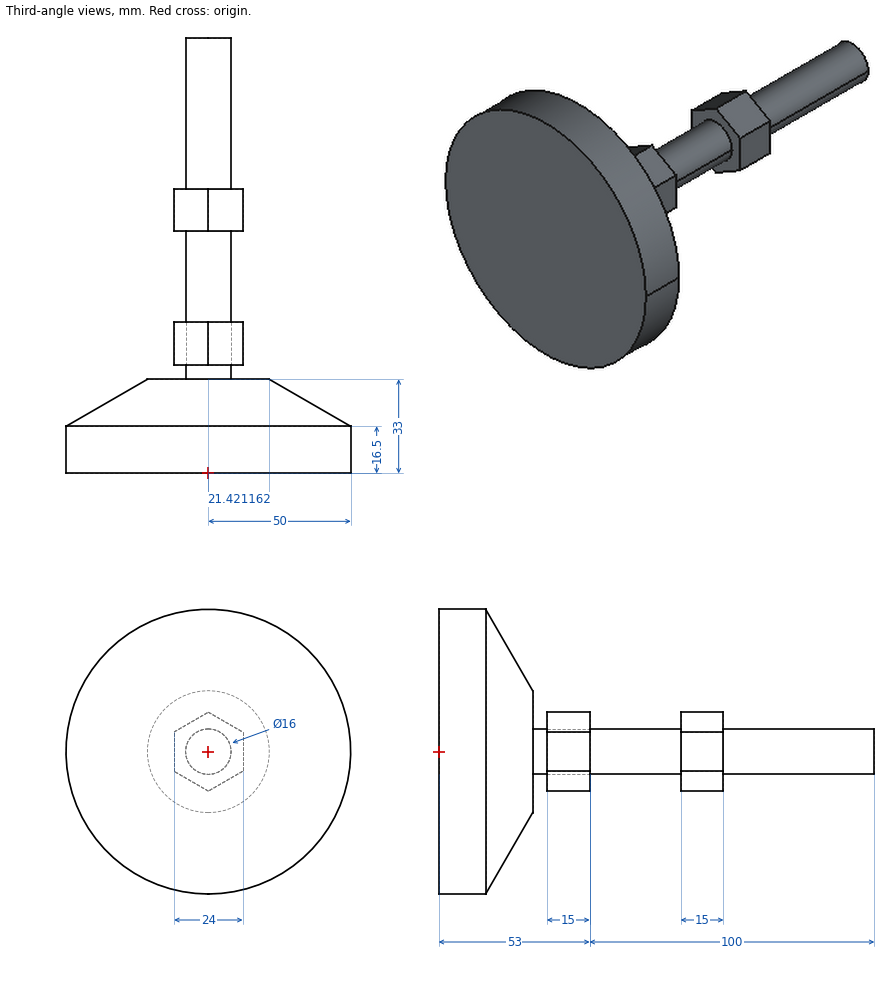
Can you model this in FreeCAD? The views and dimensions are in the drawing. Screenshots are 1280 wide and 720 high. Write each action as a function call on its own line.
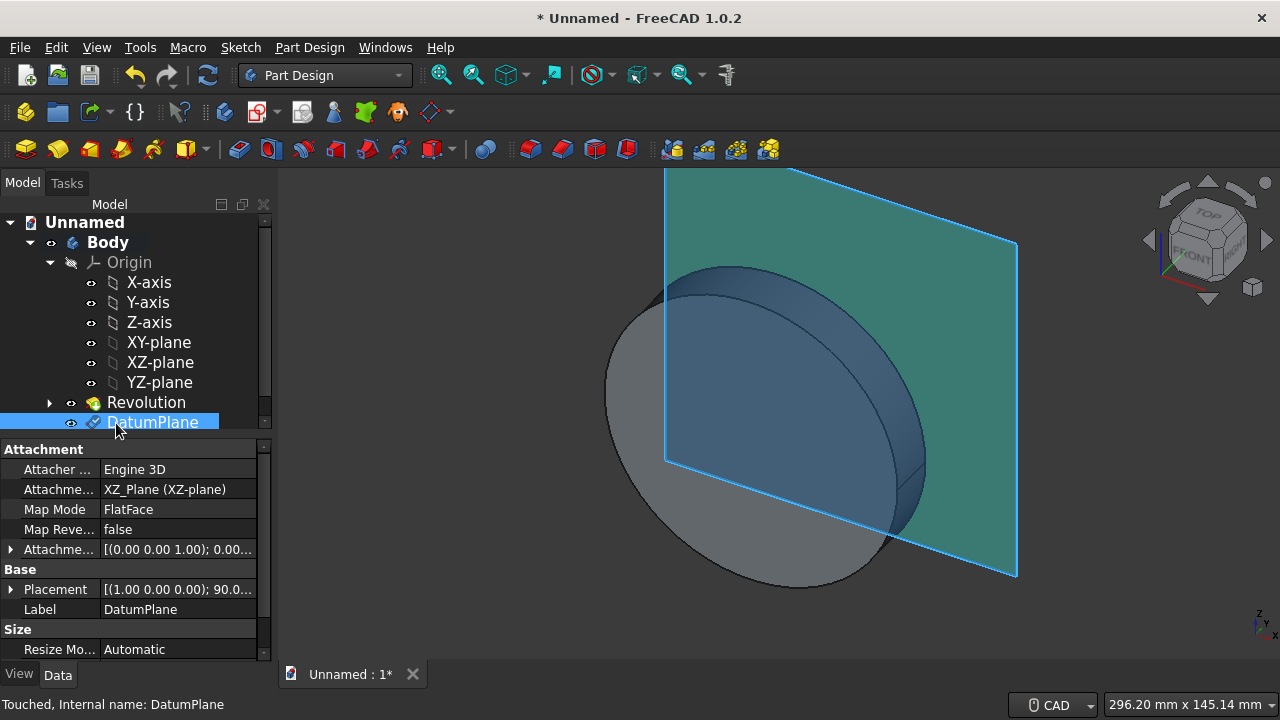
click(258, 112)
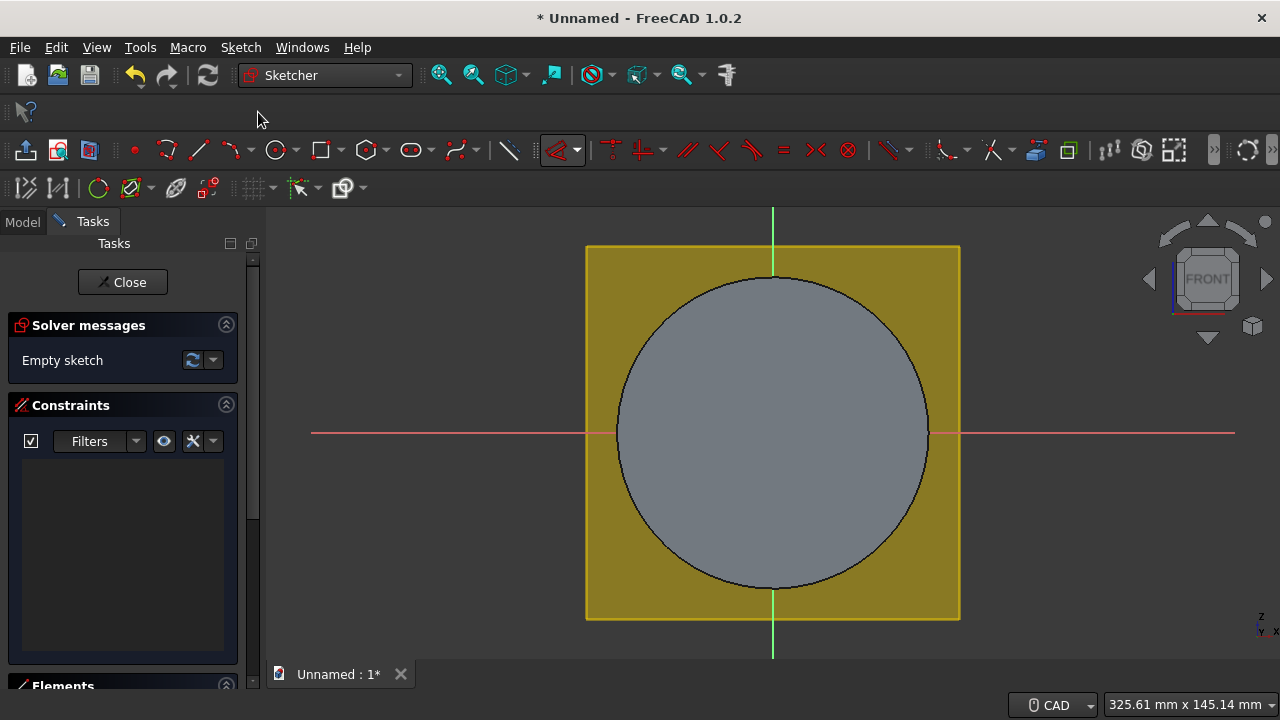
click(90, 150)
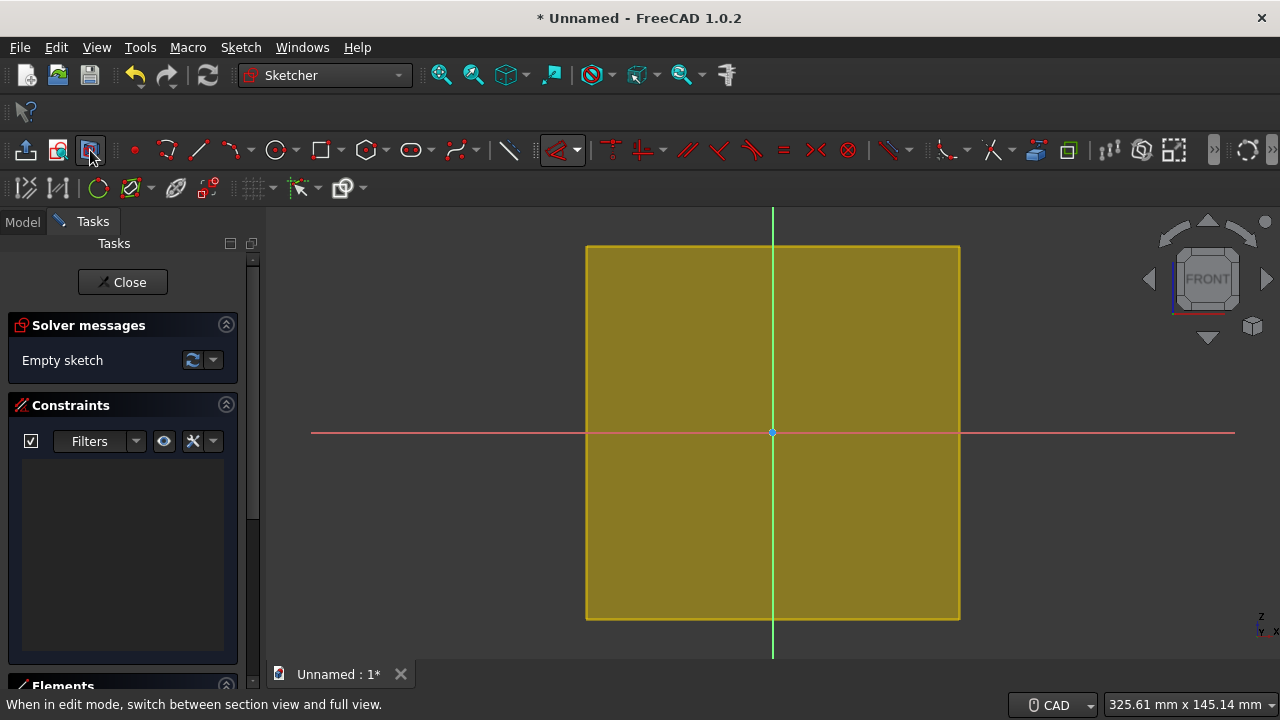
scroll(786, 433, up, 9)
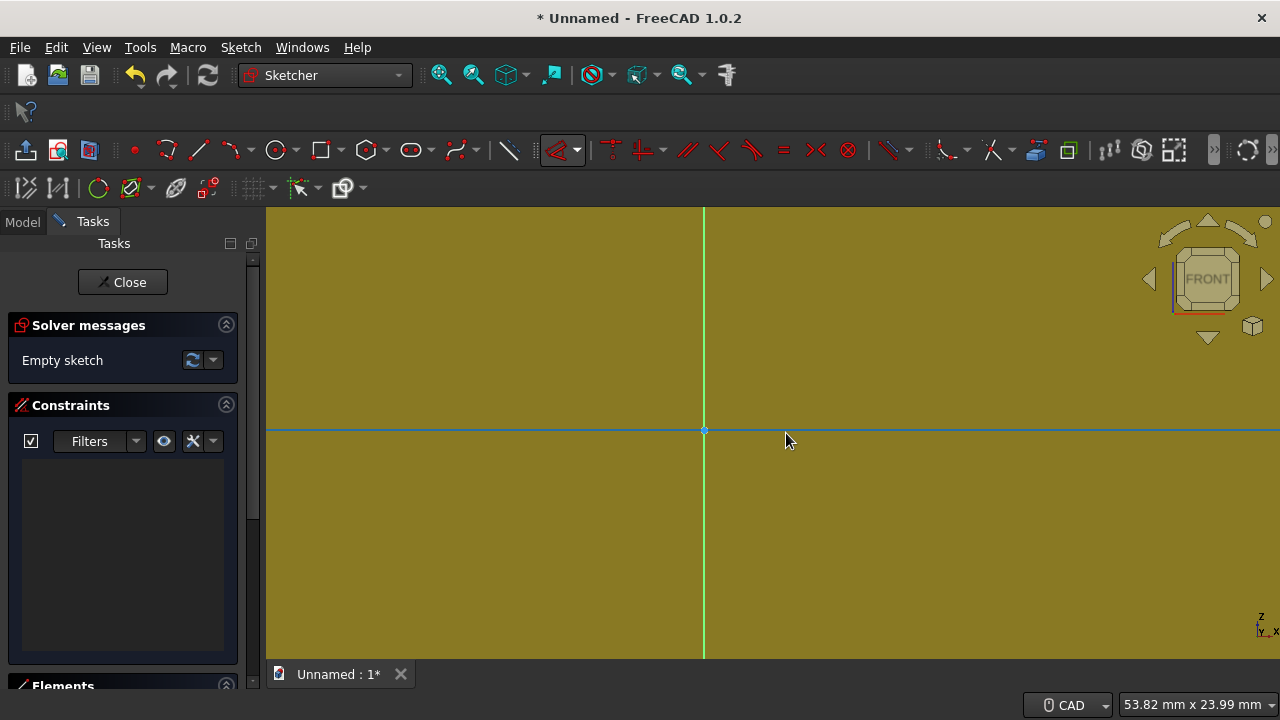
click(276, 150)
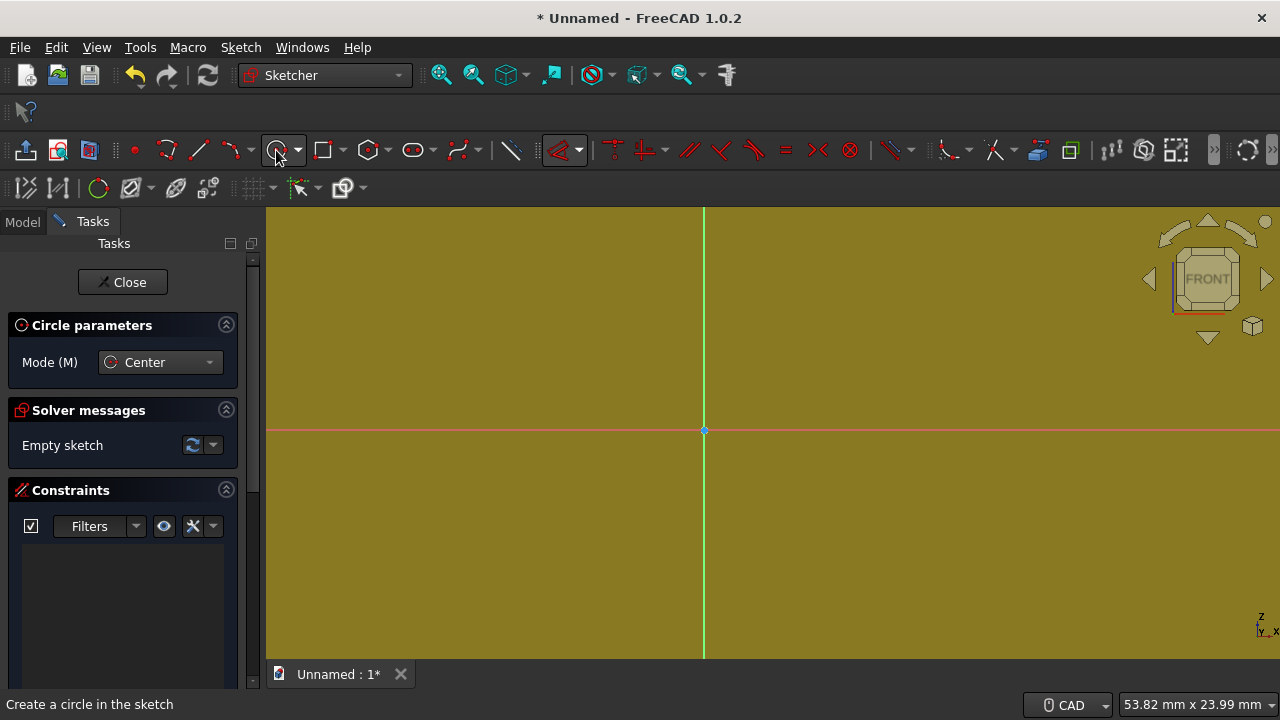
click(704, 430)
click(811, 324)
key(Escape)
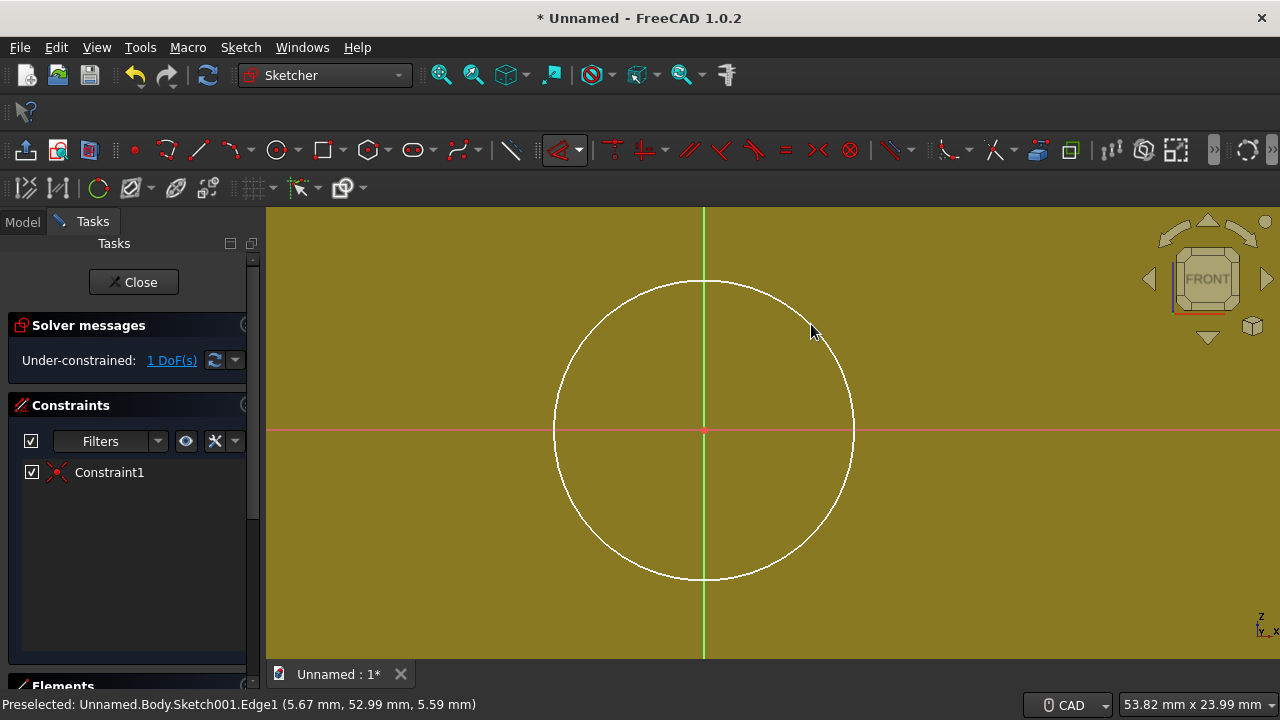
click(810, 324)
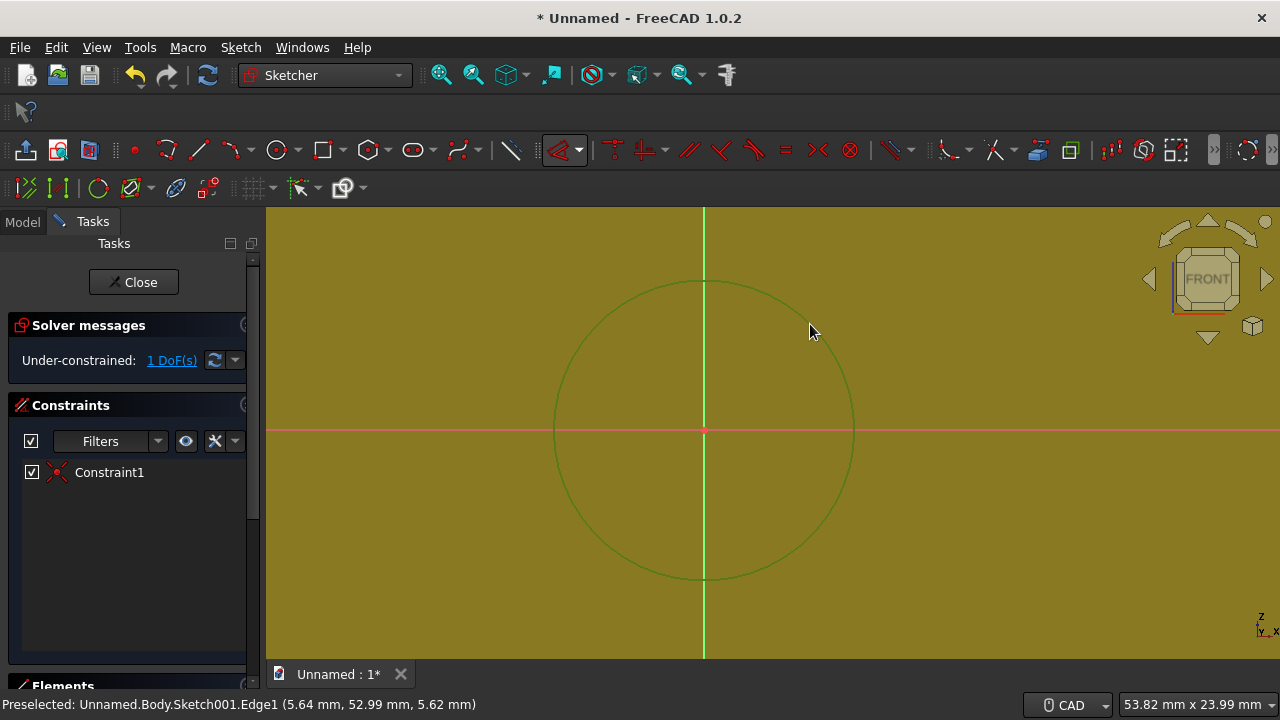
key(k)
key(o)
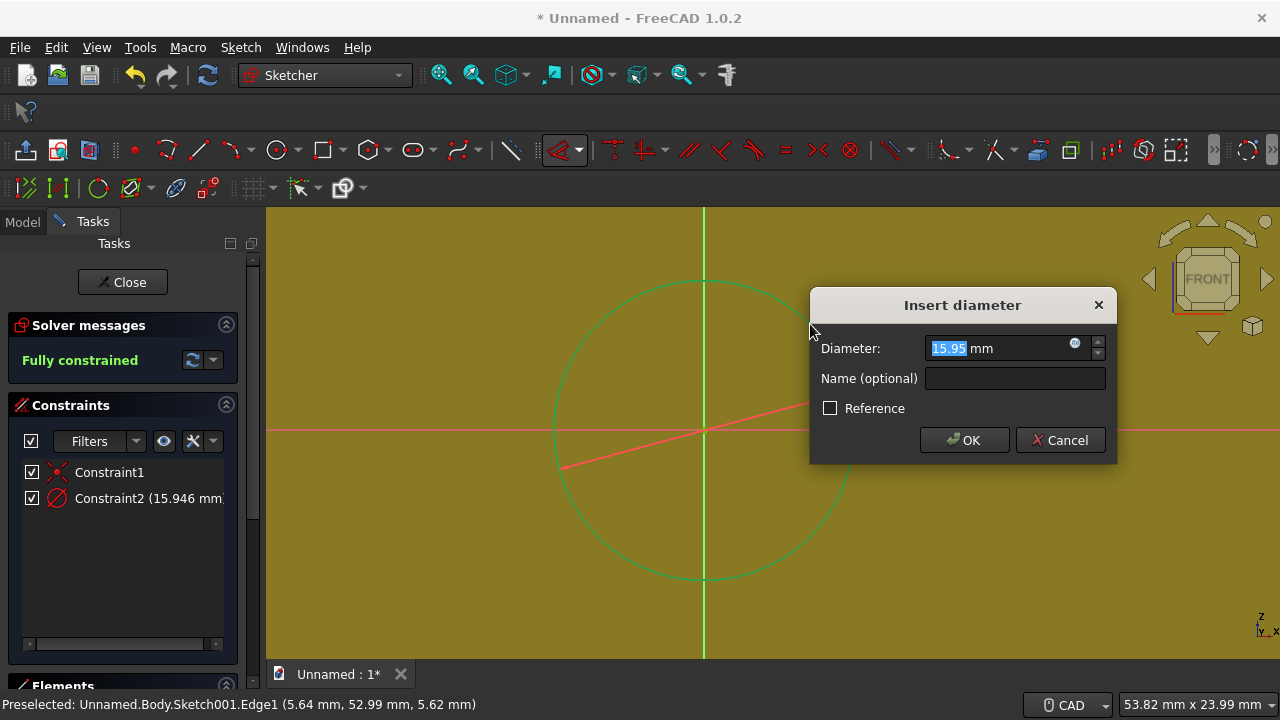
text(16)
key(Return)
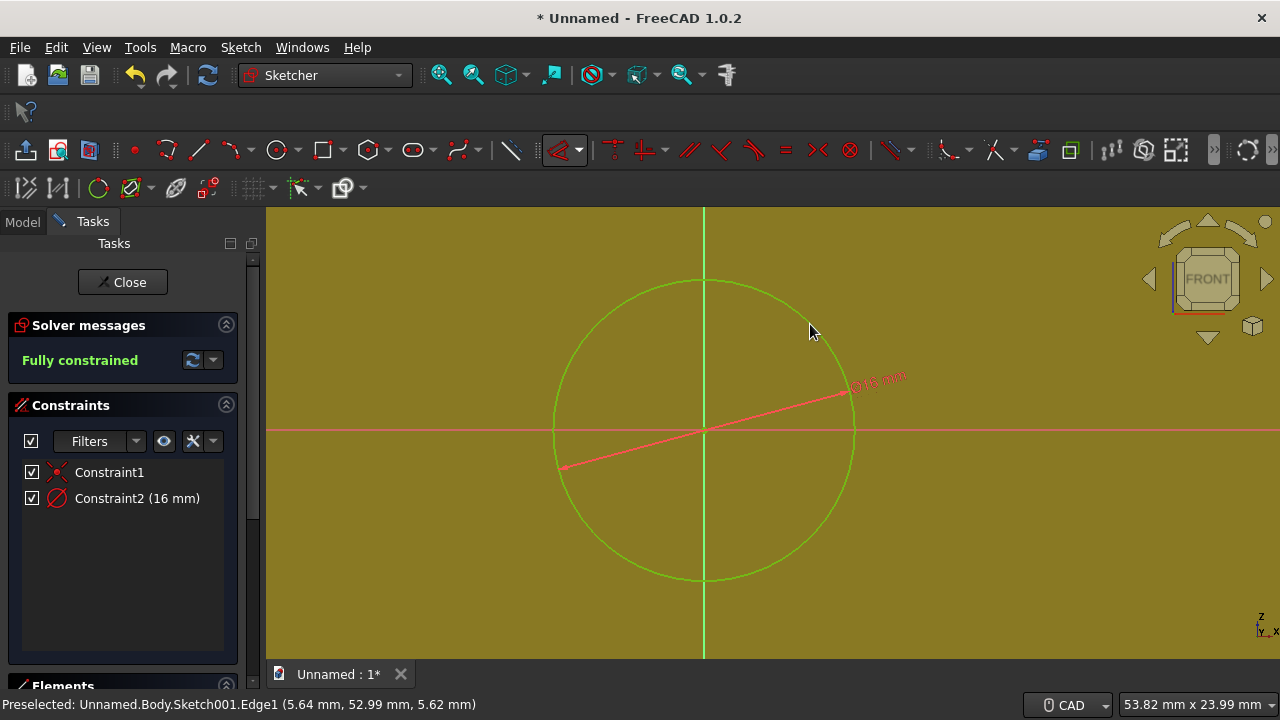
click(123, 282)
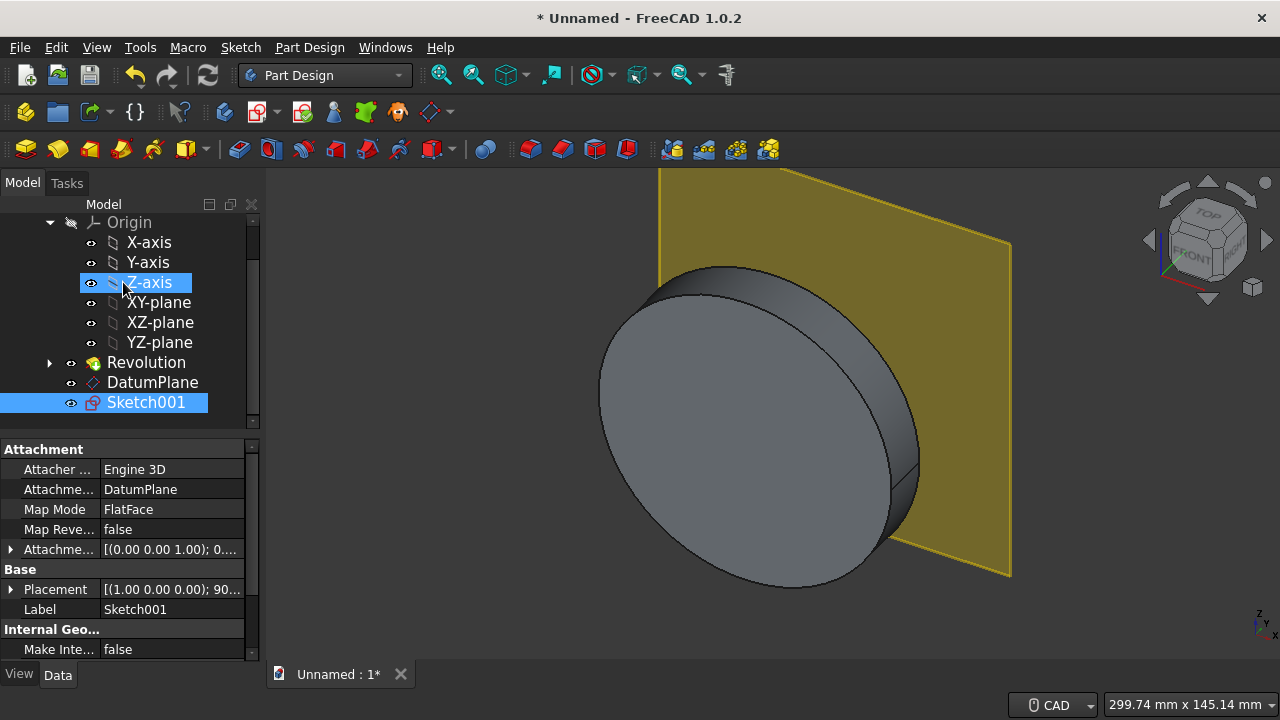
click(26, 150)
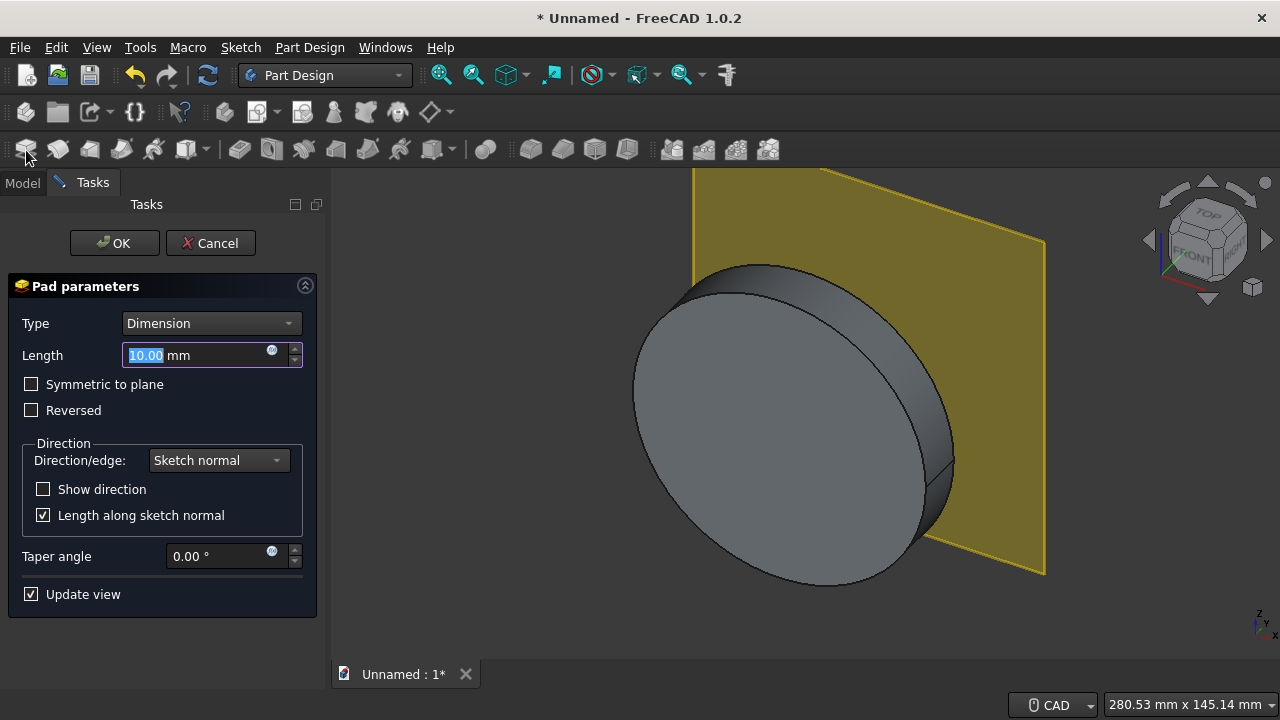
click(212, 324)